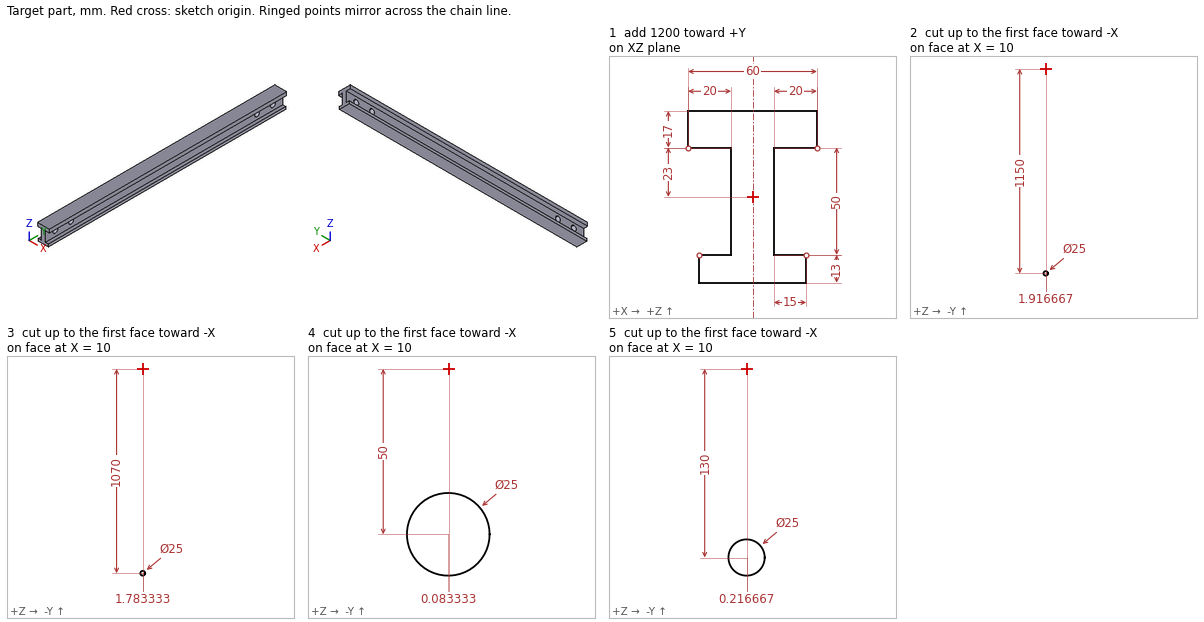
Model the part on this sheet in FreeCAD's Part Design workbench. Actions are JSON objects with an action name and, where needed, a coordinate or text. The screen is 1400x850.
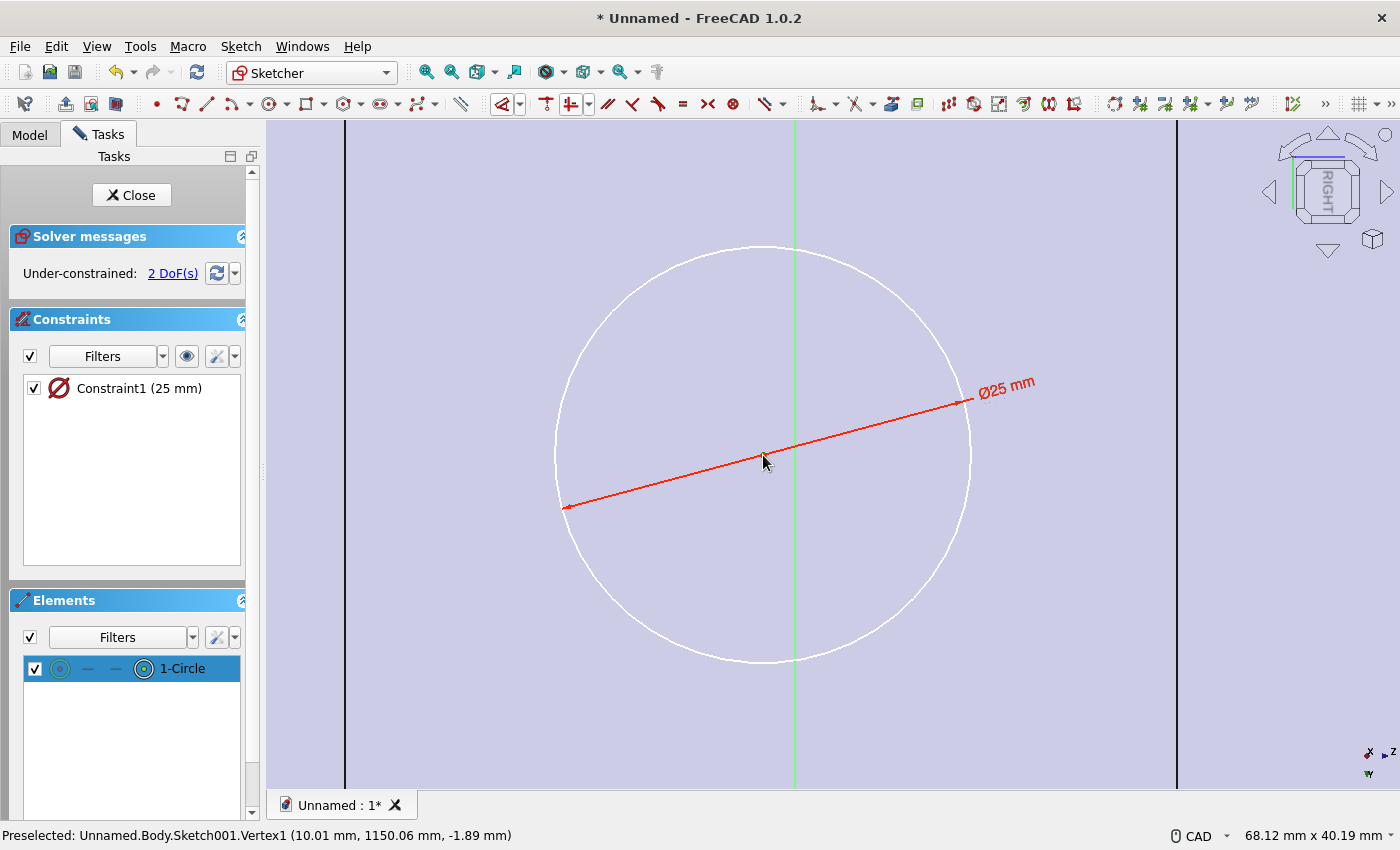
{"action": "key", "text": "i"}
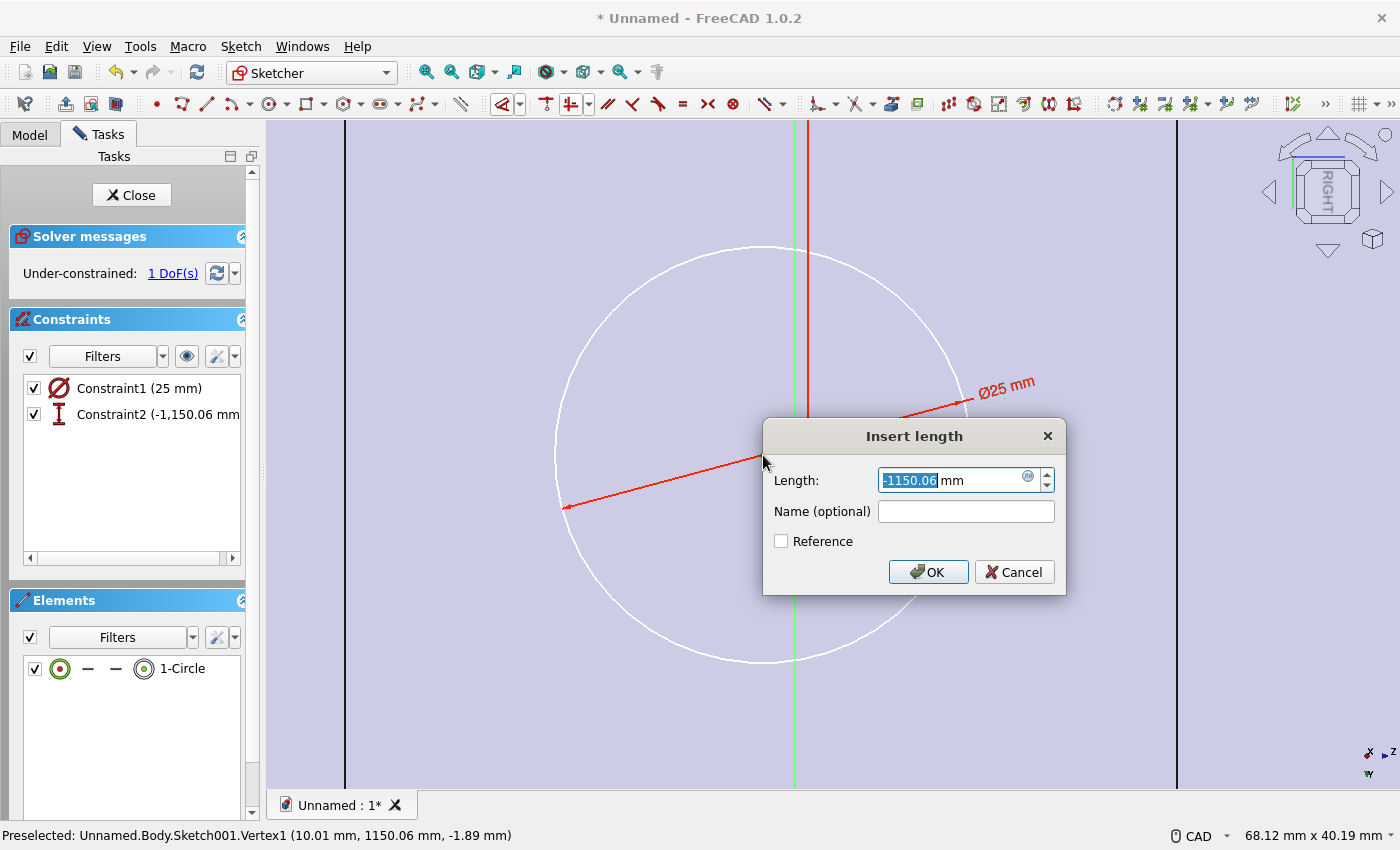
{"action": "type", "text": "-1150"}
{"action": "key", "text": "Return"}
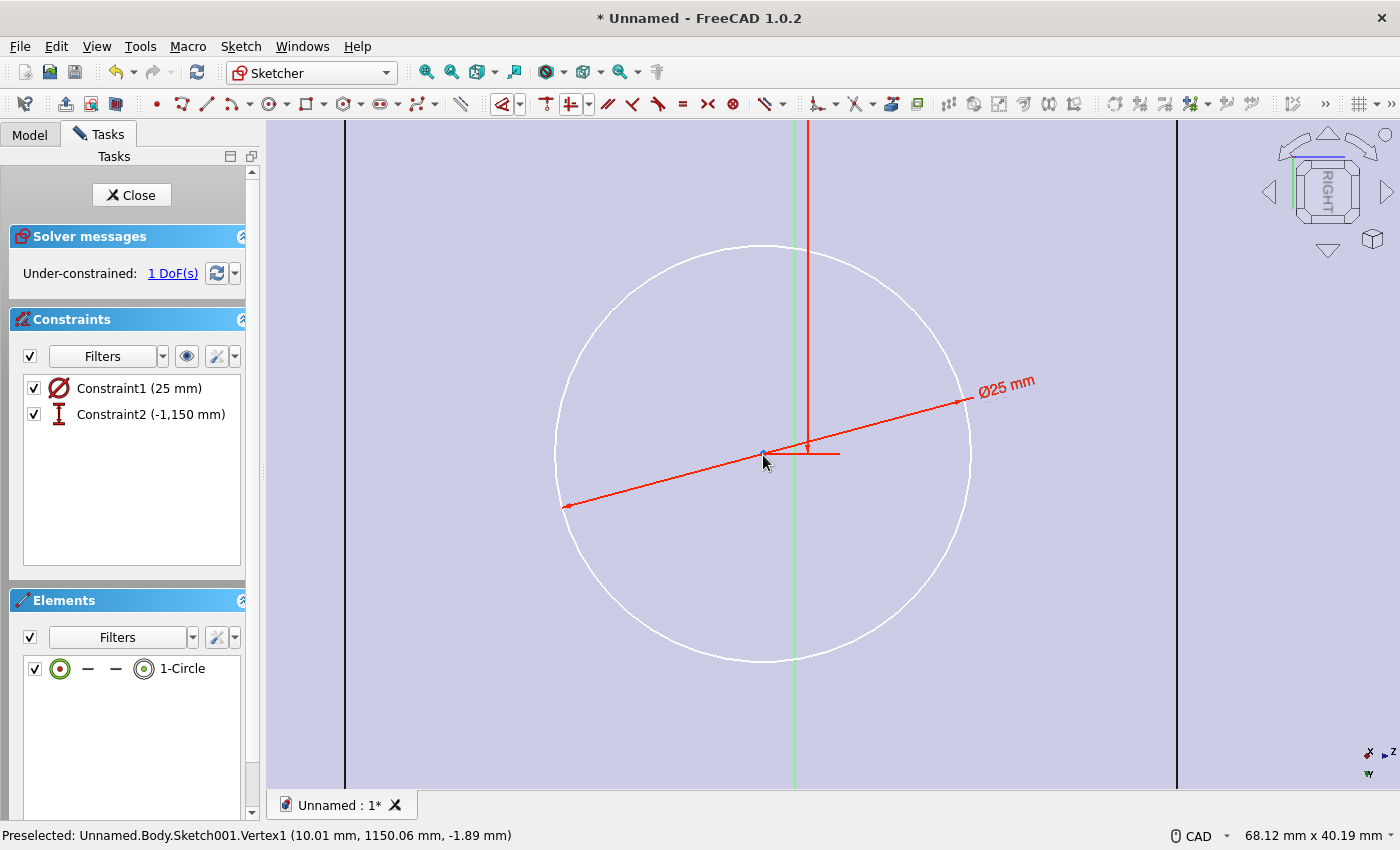
{"action": "scroll", "coordinate": [763, 454], "scroll_direction": "up", "scroll_amount": 2}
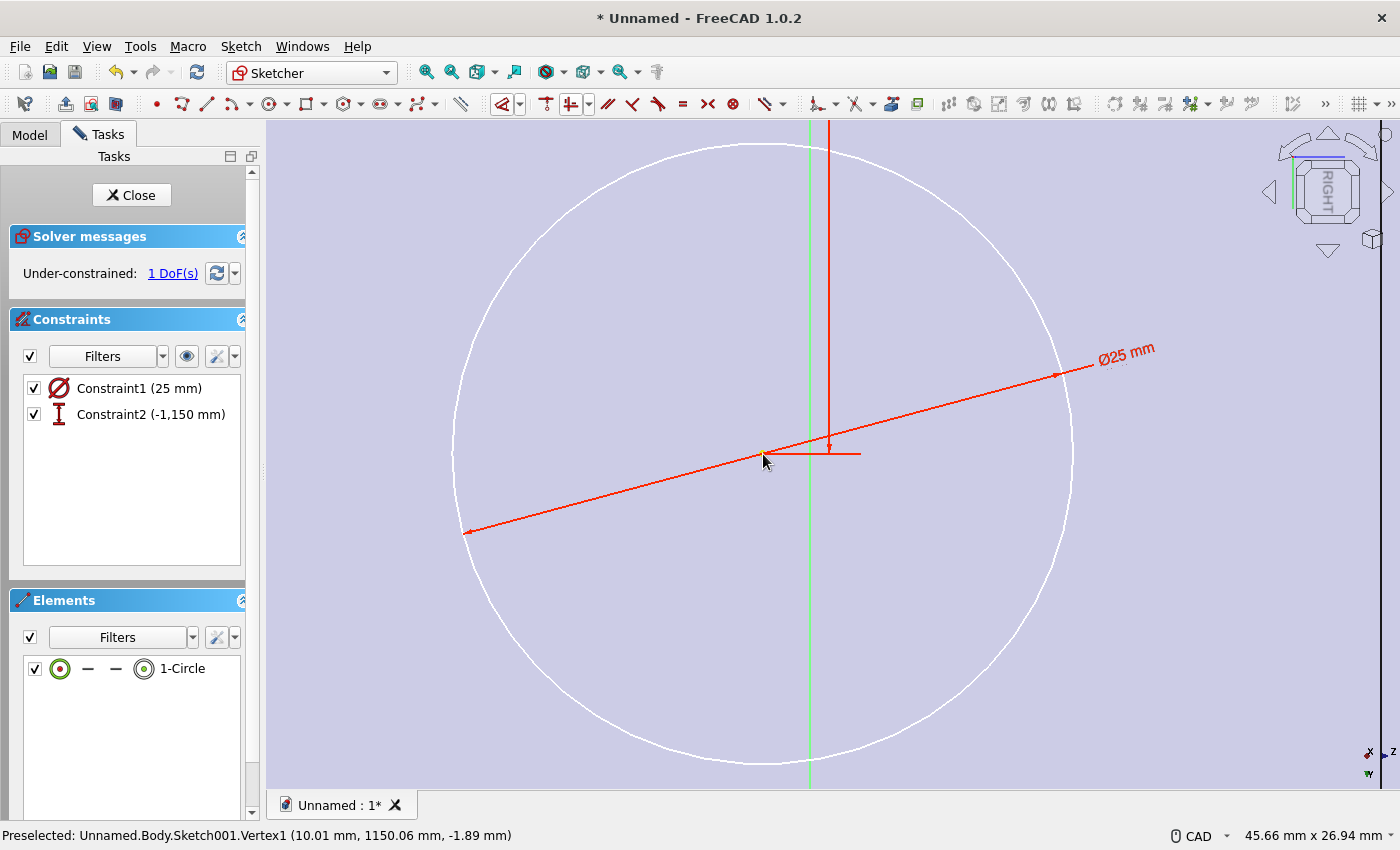
{"action": "left_click", "coordinate": [763, 454]}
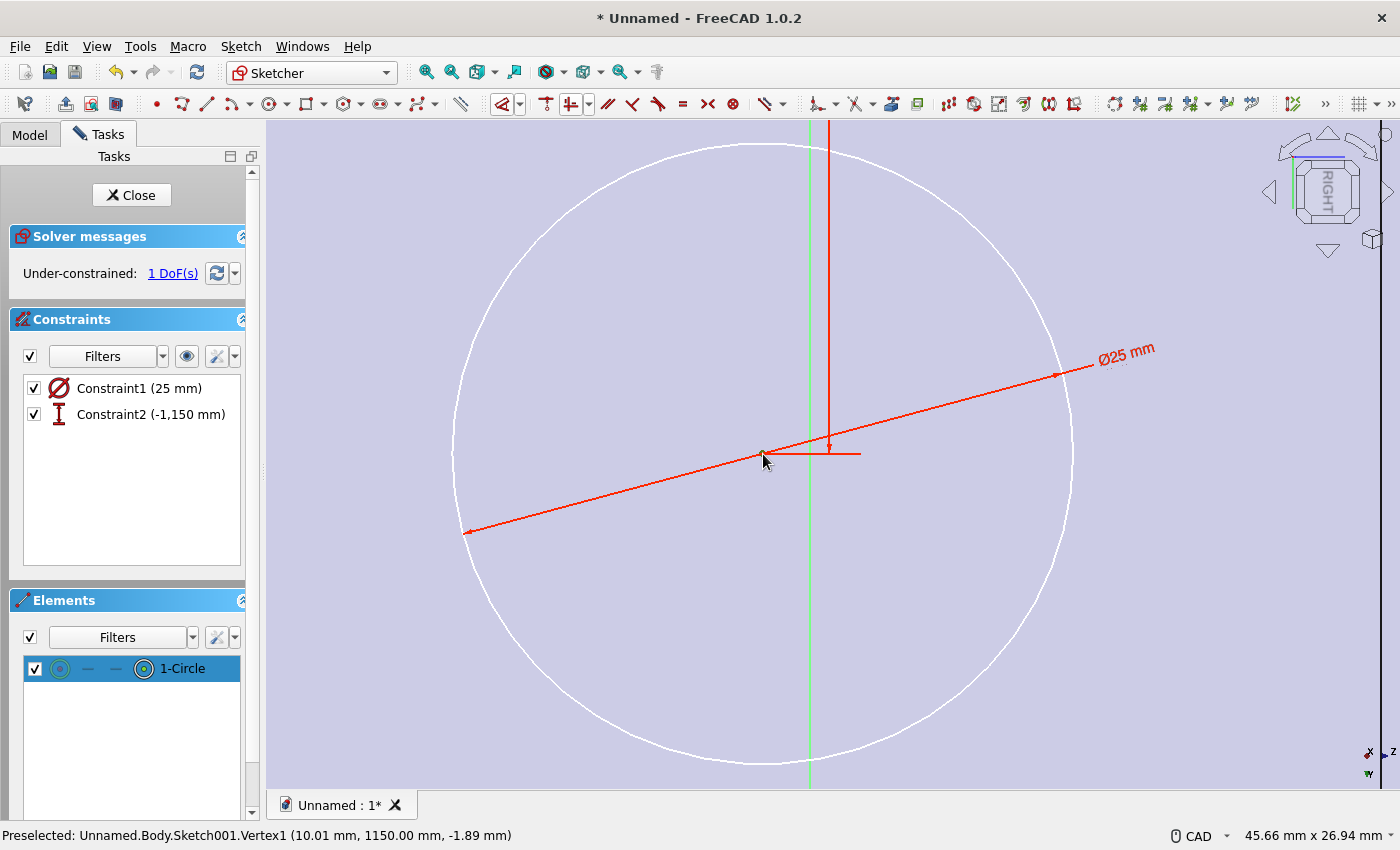
{"action": "key", "text": "l"}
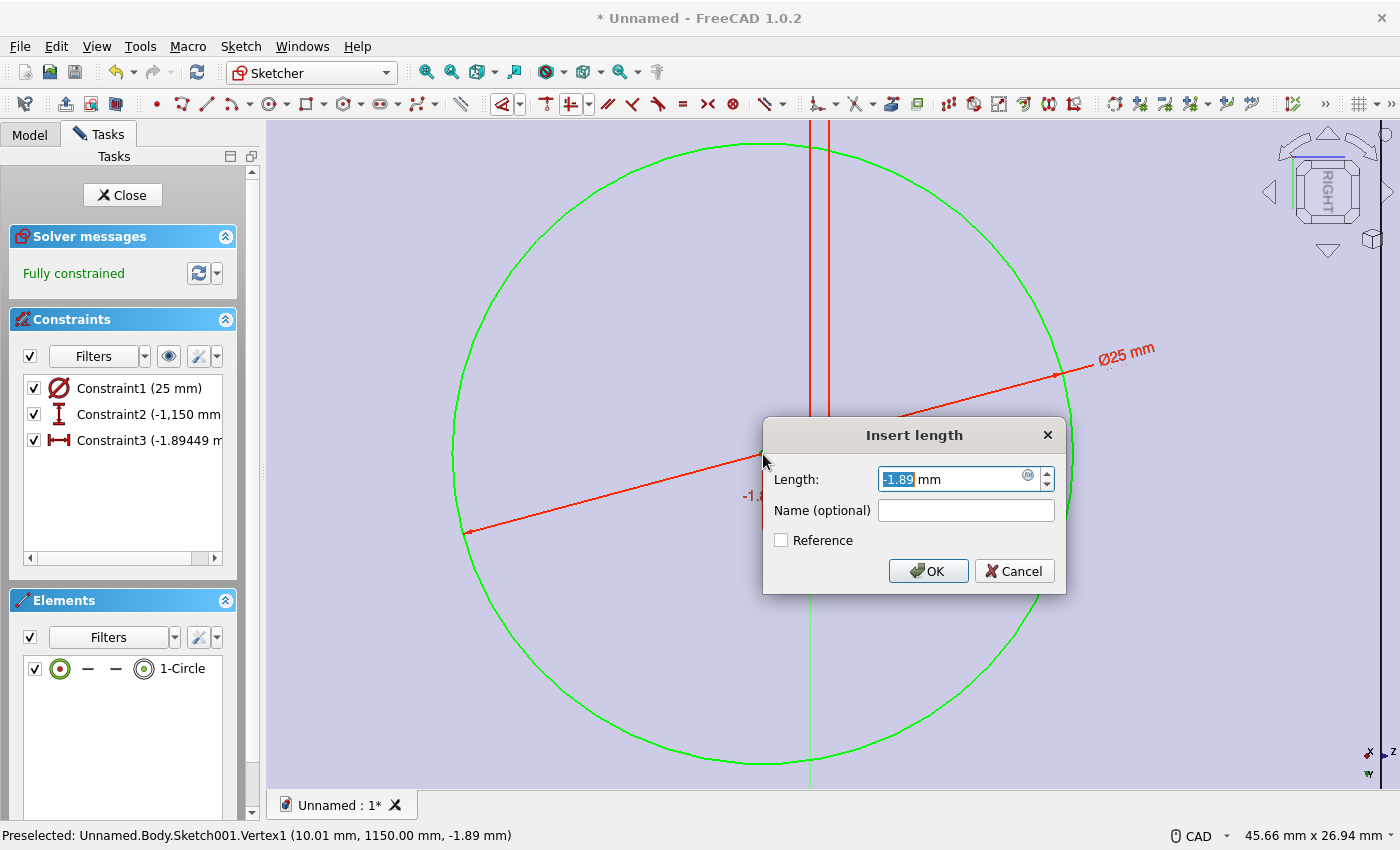
{"action": "type", "text": "-1.916667"}
{"action": "key", "text": "Return"}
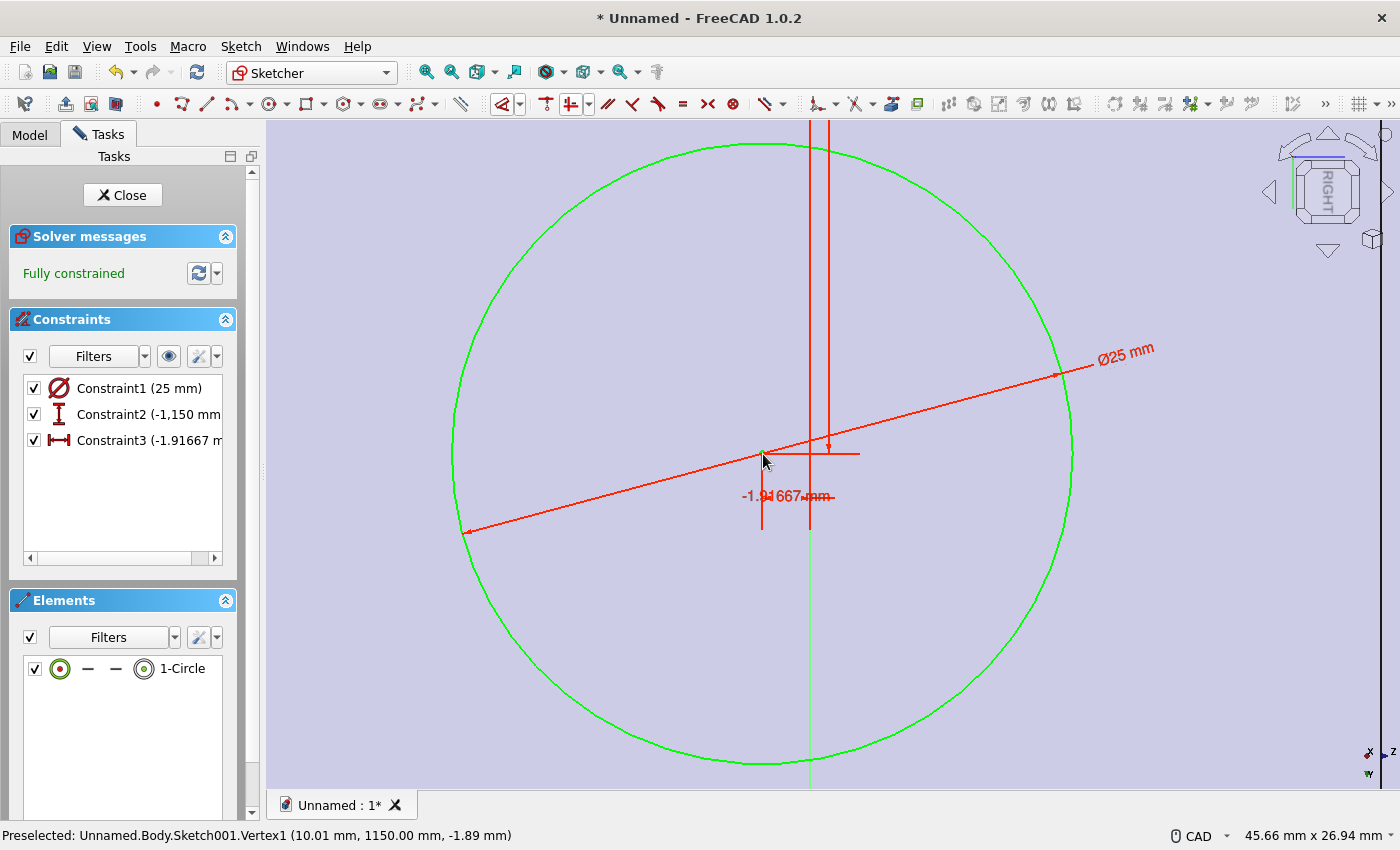
{"action": "left_click", "coordinate": [123, 195]}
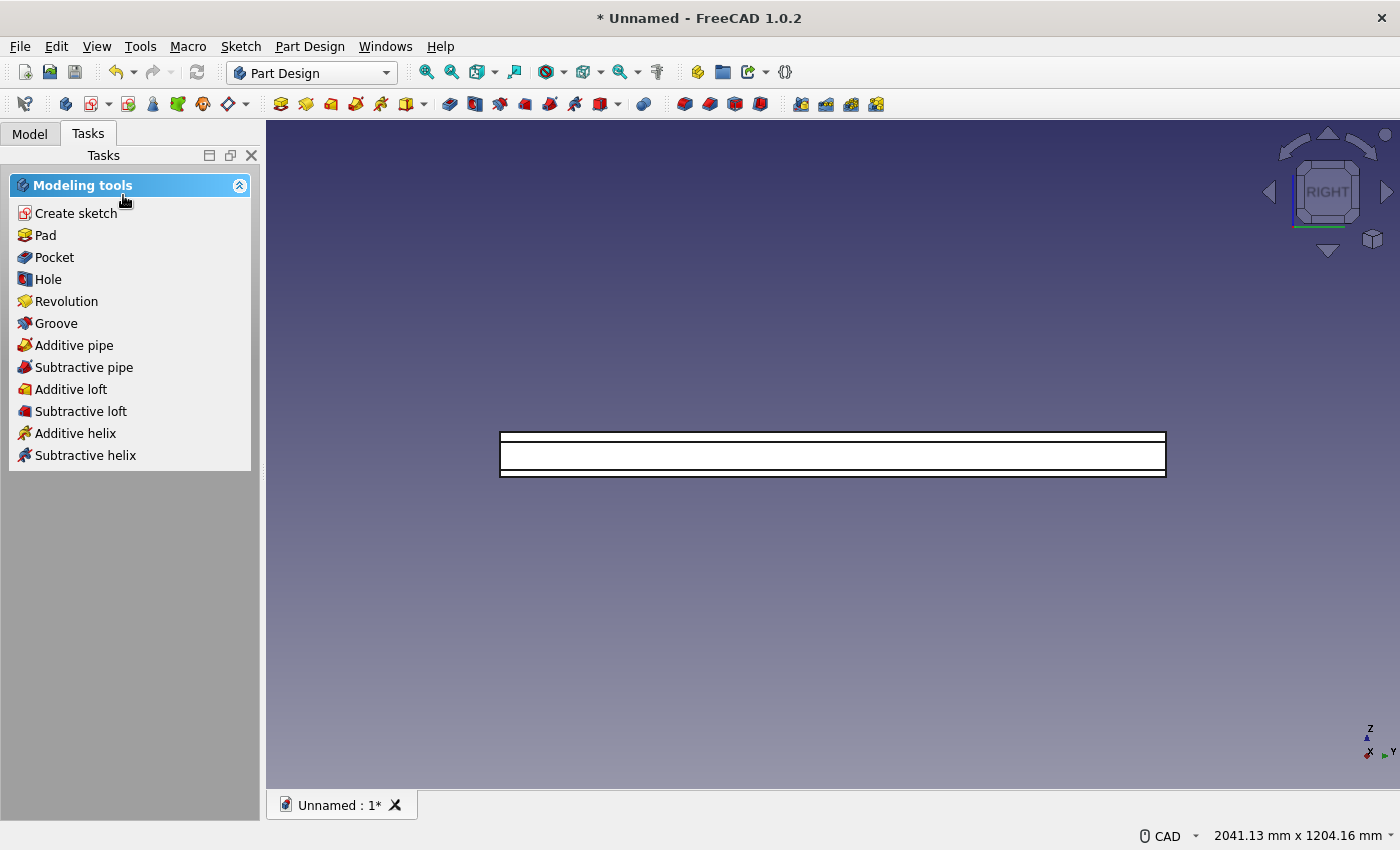
{"action": "left_click", "coordinate": [450, 104]}